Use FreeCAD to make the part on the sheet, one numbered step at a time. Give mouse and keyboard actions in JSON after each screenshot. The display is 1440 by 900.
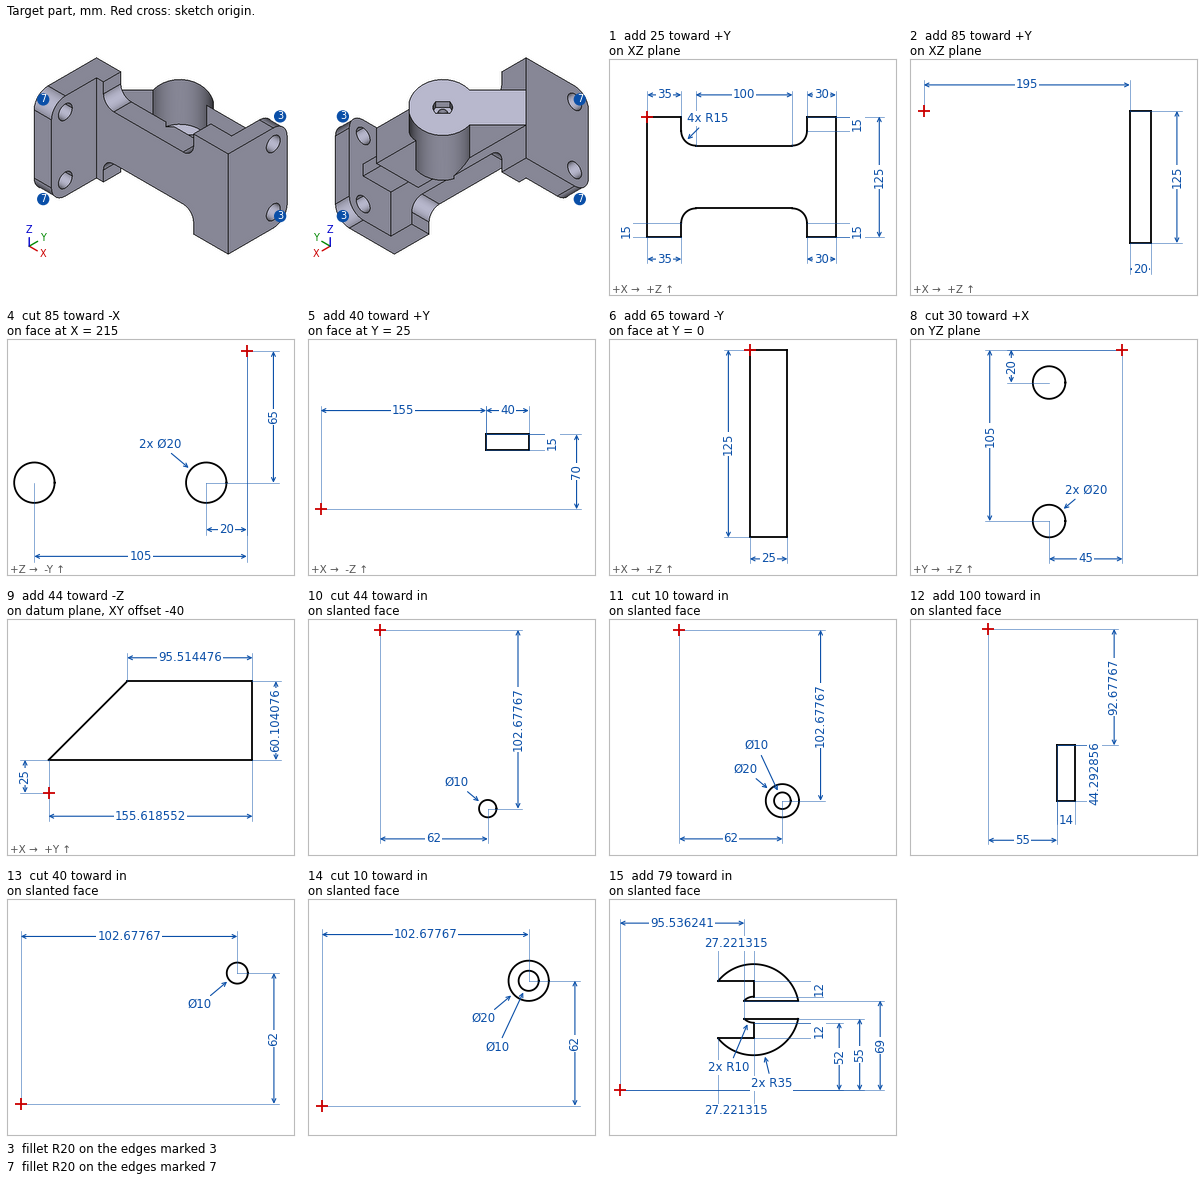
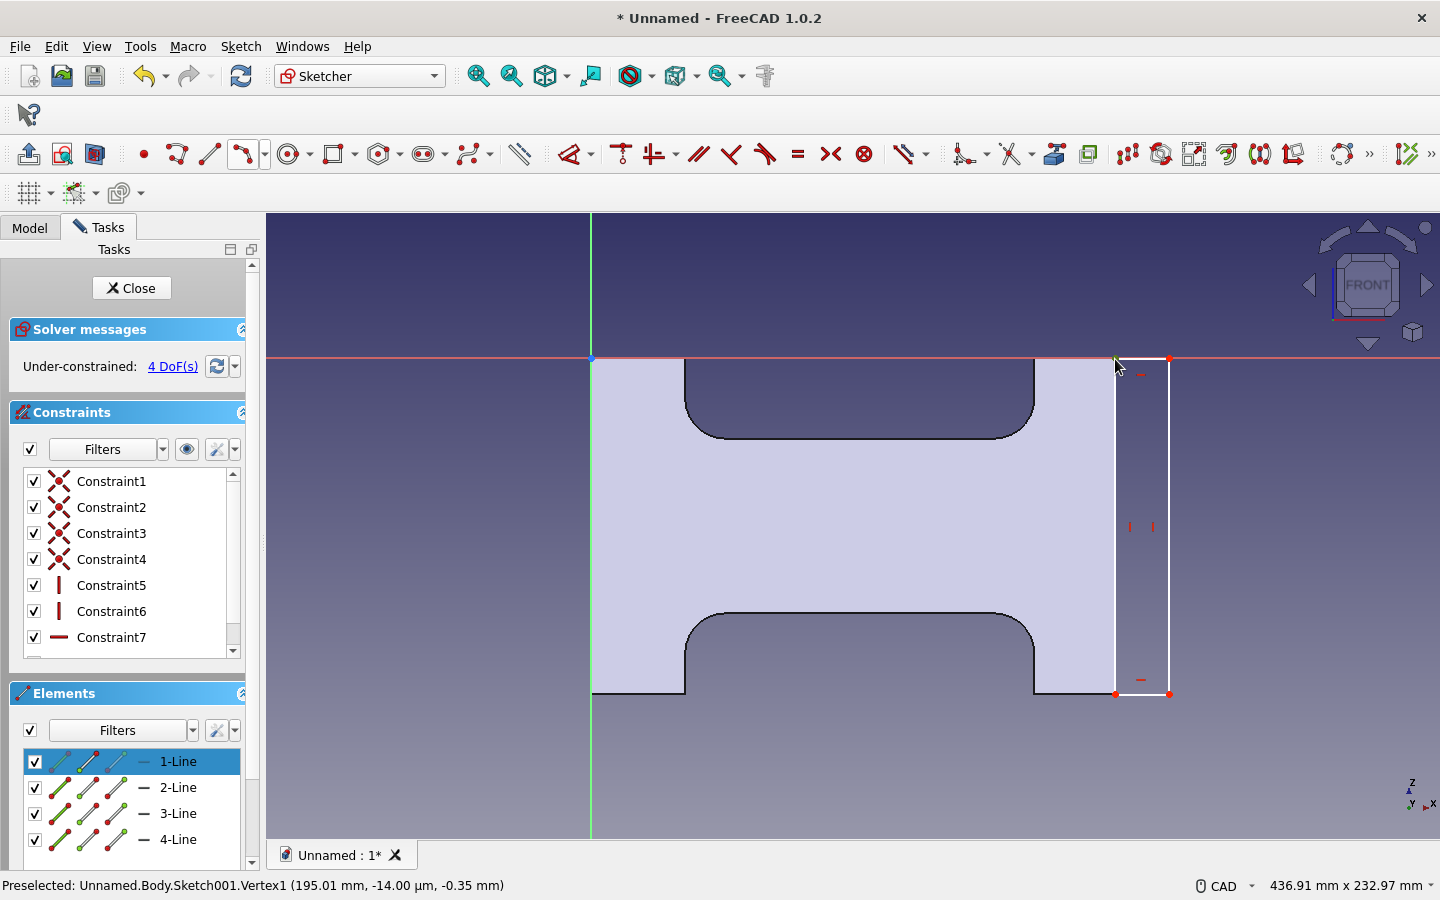
{"action": "left_click", "coordinate": [364, 358]}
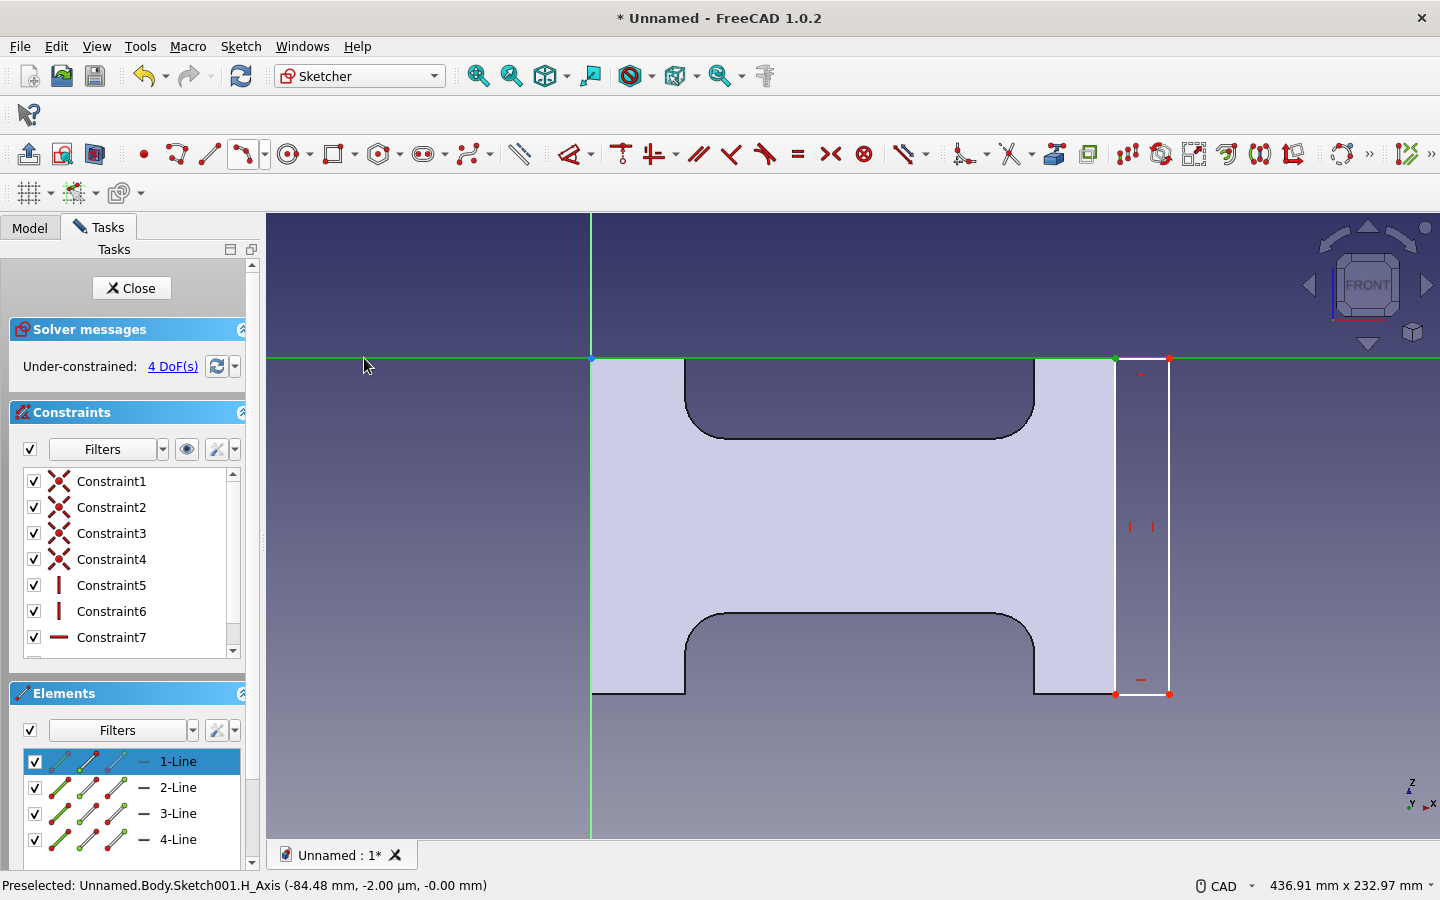
{"action": "left_click", "coordinate": [621, 154]}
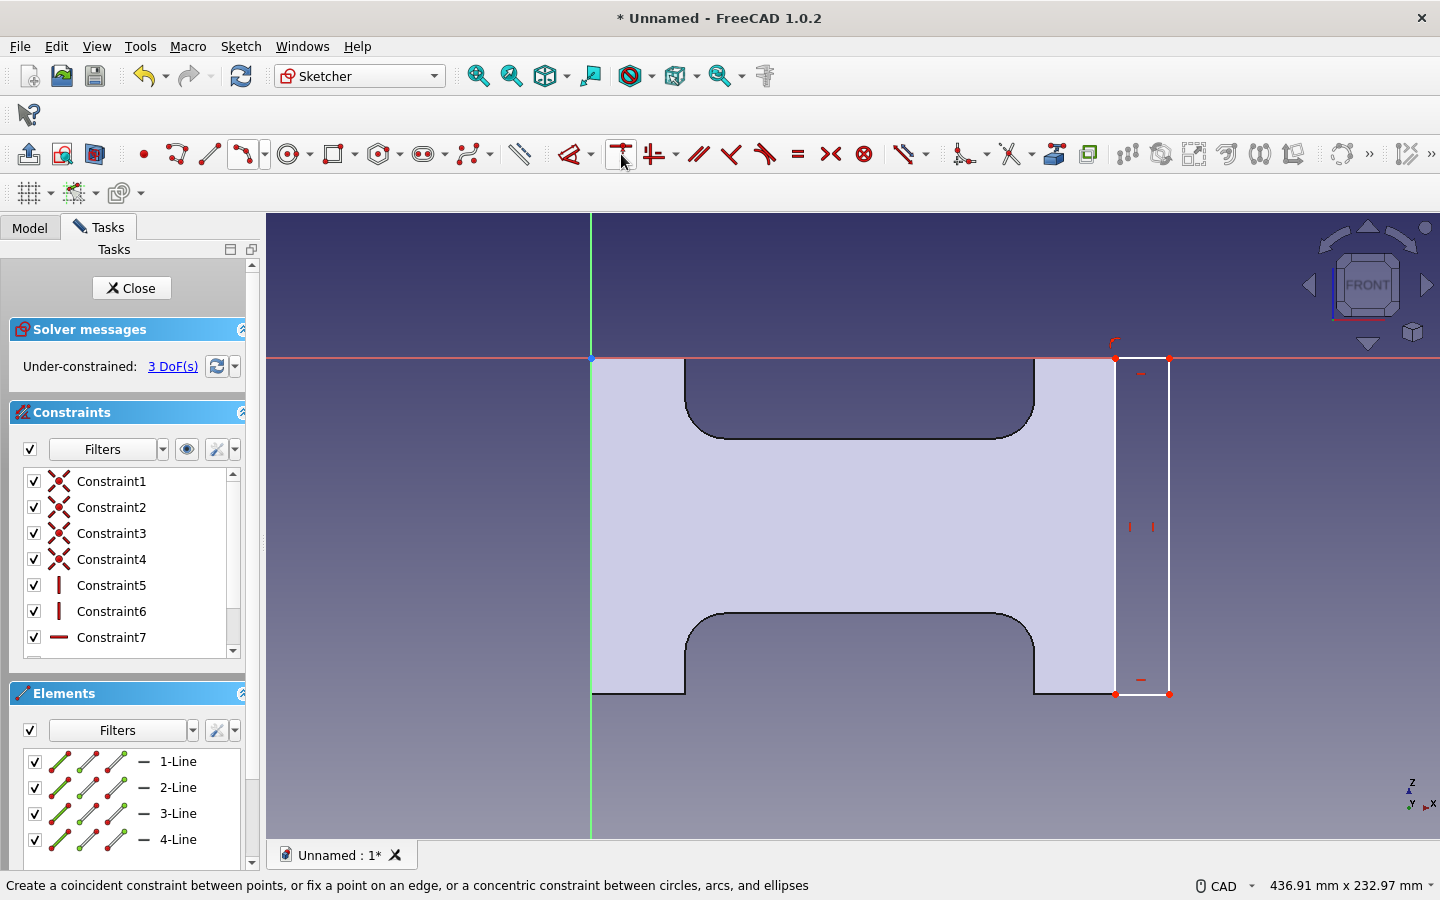
{"action": "left_click", "coordinate": [568, 154]}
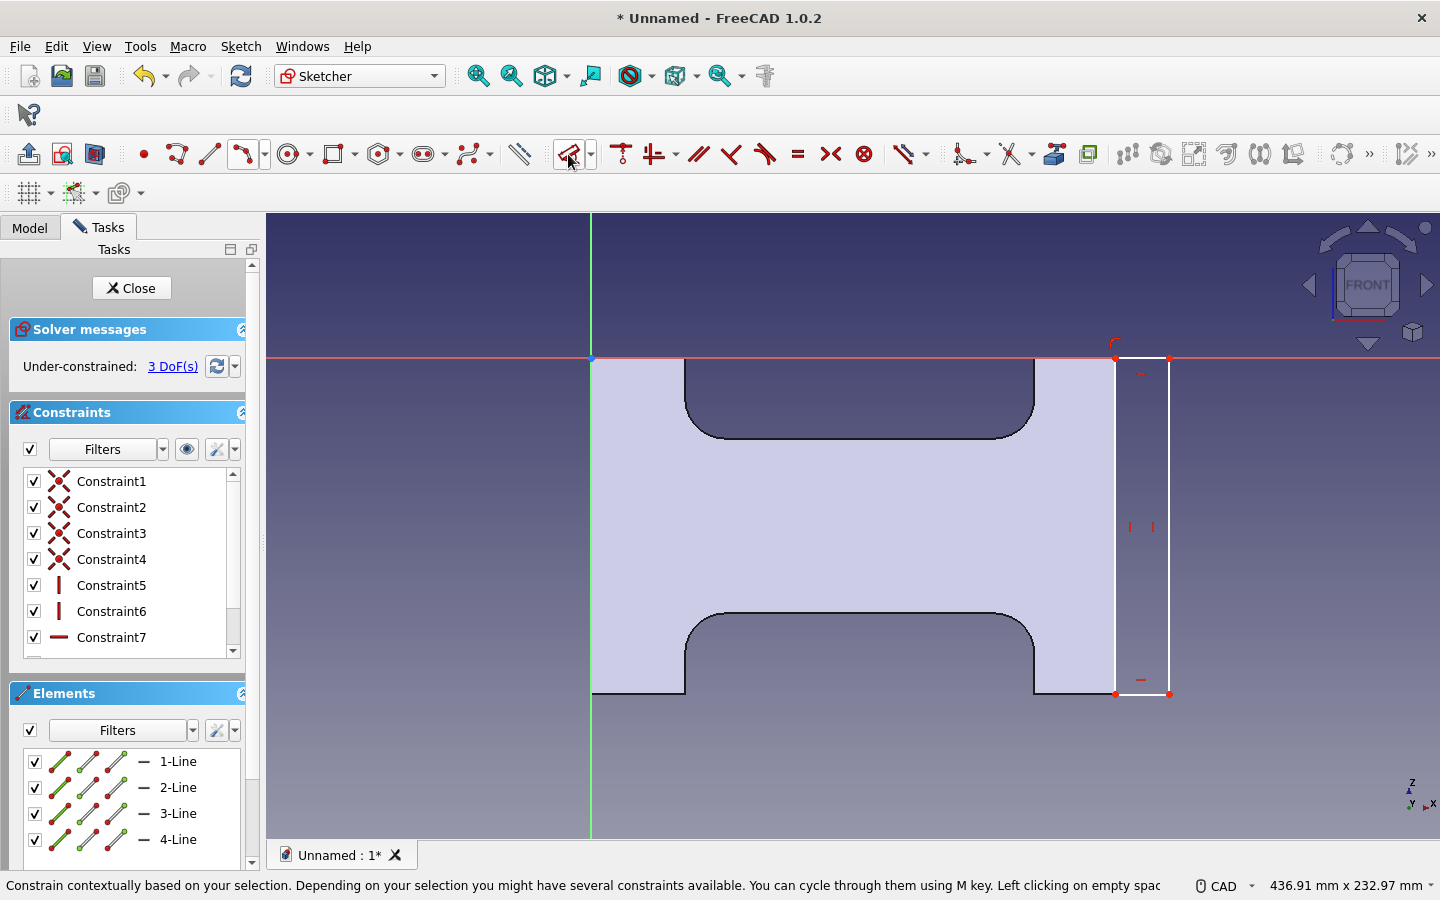
{"action": "left_click", "coordinate": [1131, 695]}
{"action": "left_click", "coordinate": [1142, 729]}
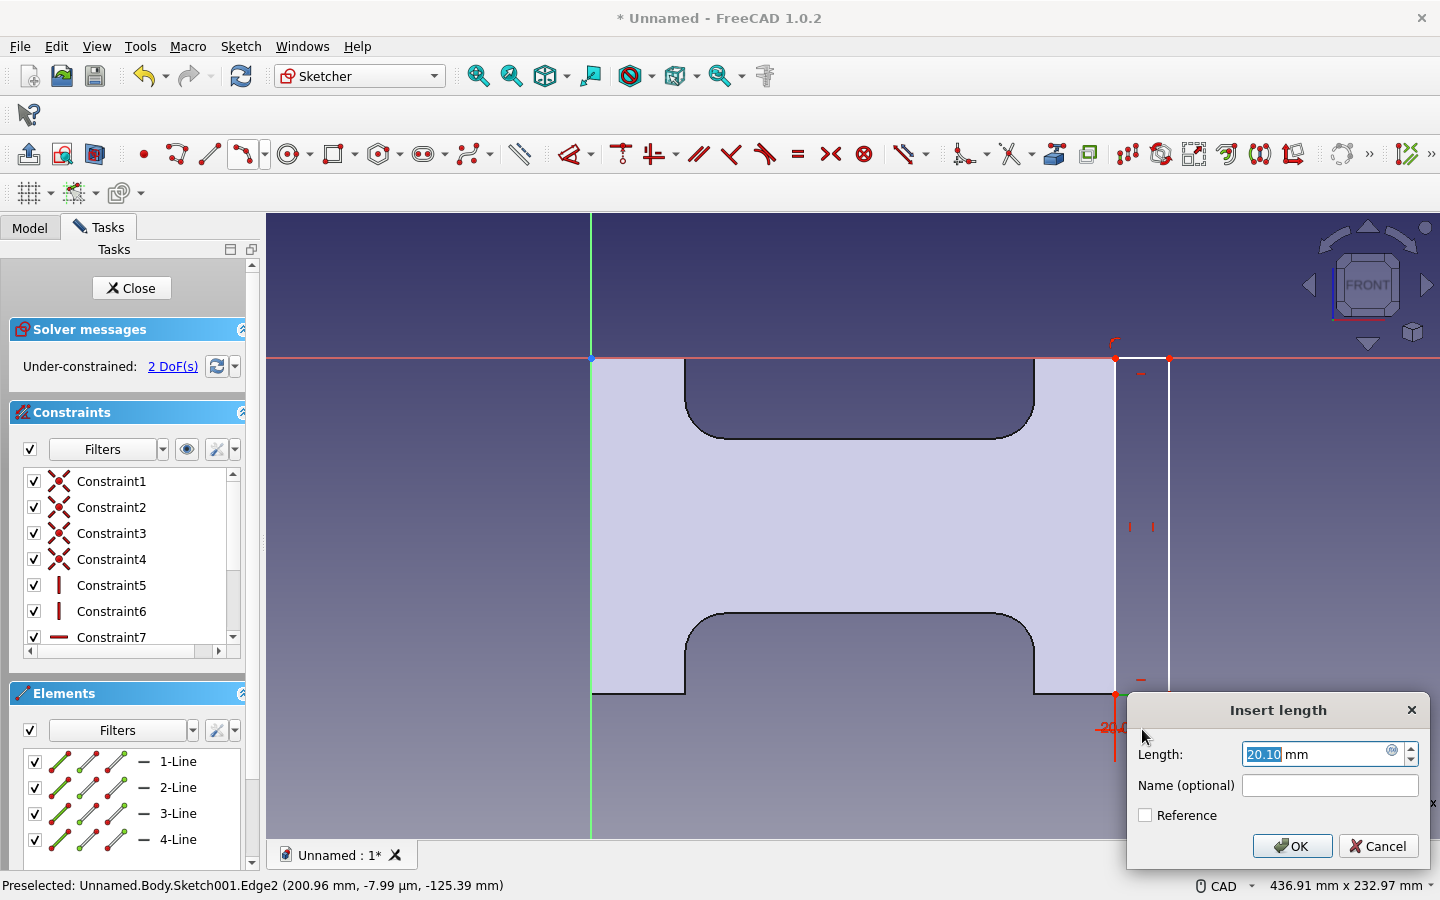
{"action": "type", "text": "20"}
{"action": "key", "text": "Return"}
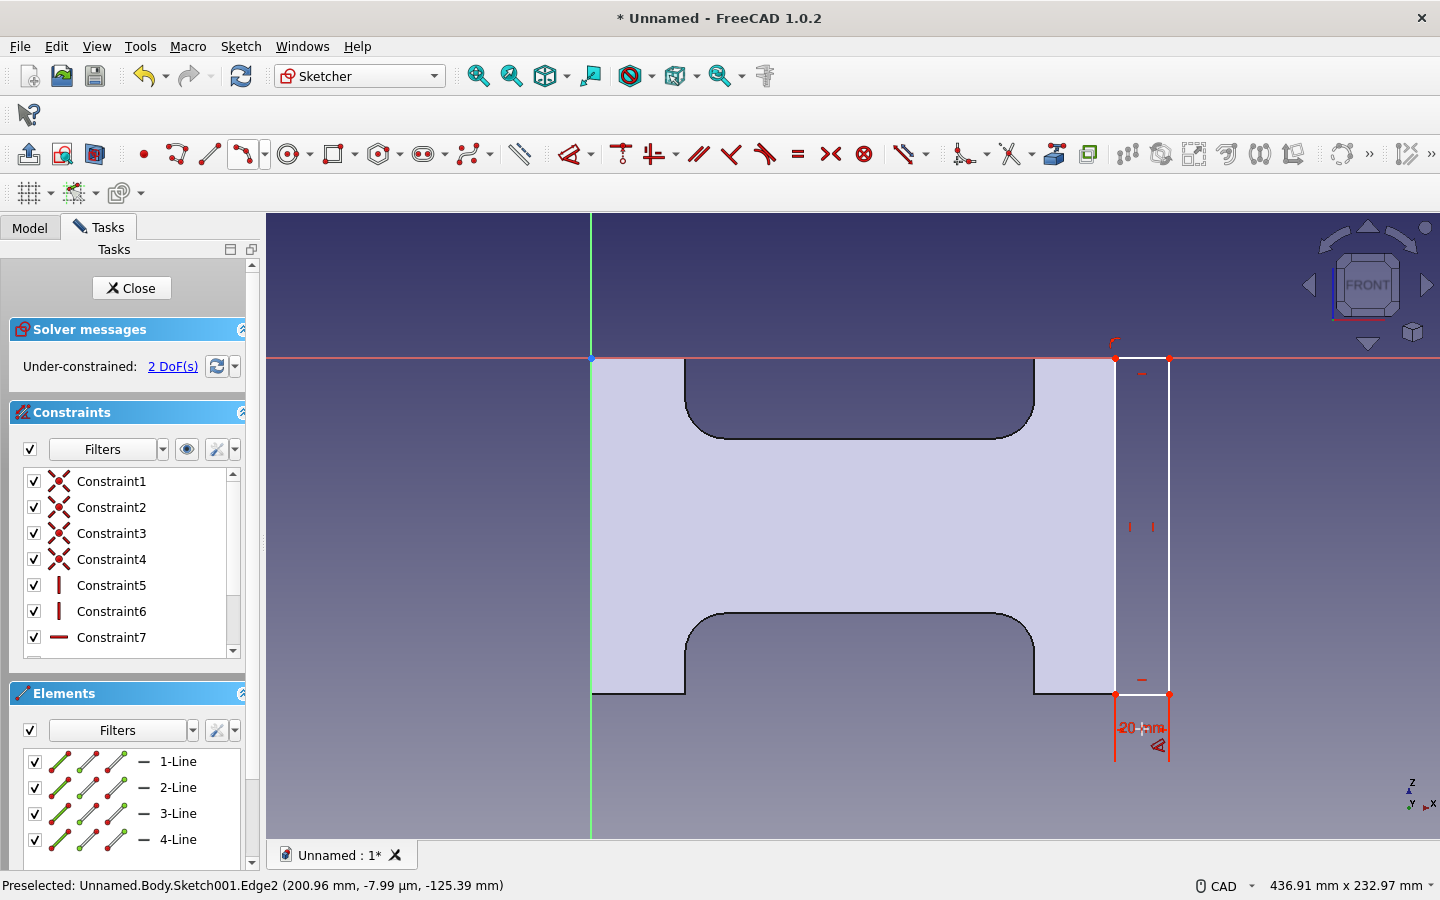
{"action": "left_click", "coordinate": [1115, 459]}
{"action": "left_click", "coordinate": [1149, 527]}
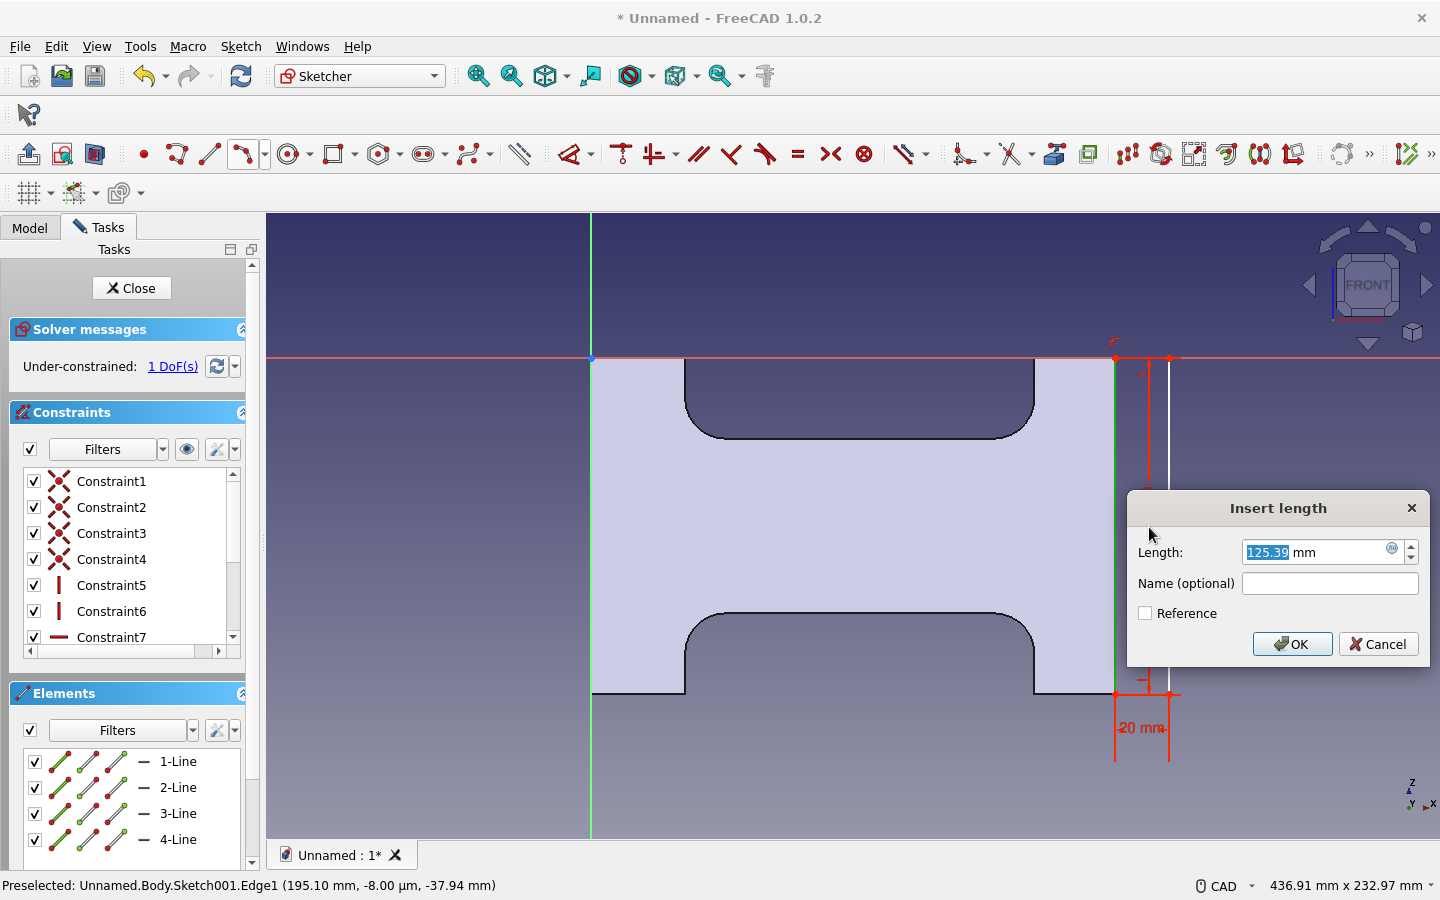
{"action": "type", "text": "125"}
{"action": "key", "text": "Return"}